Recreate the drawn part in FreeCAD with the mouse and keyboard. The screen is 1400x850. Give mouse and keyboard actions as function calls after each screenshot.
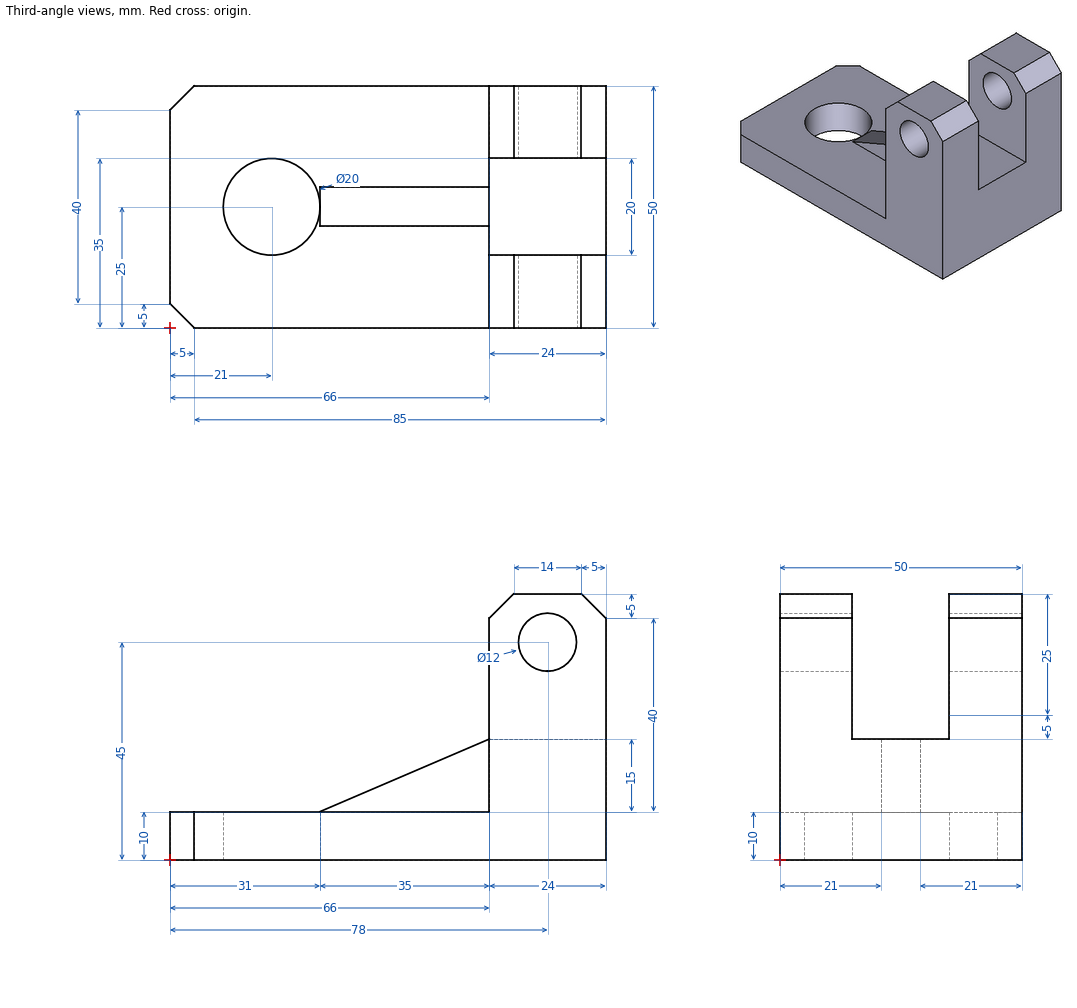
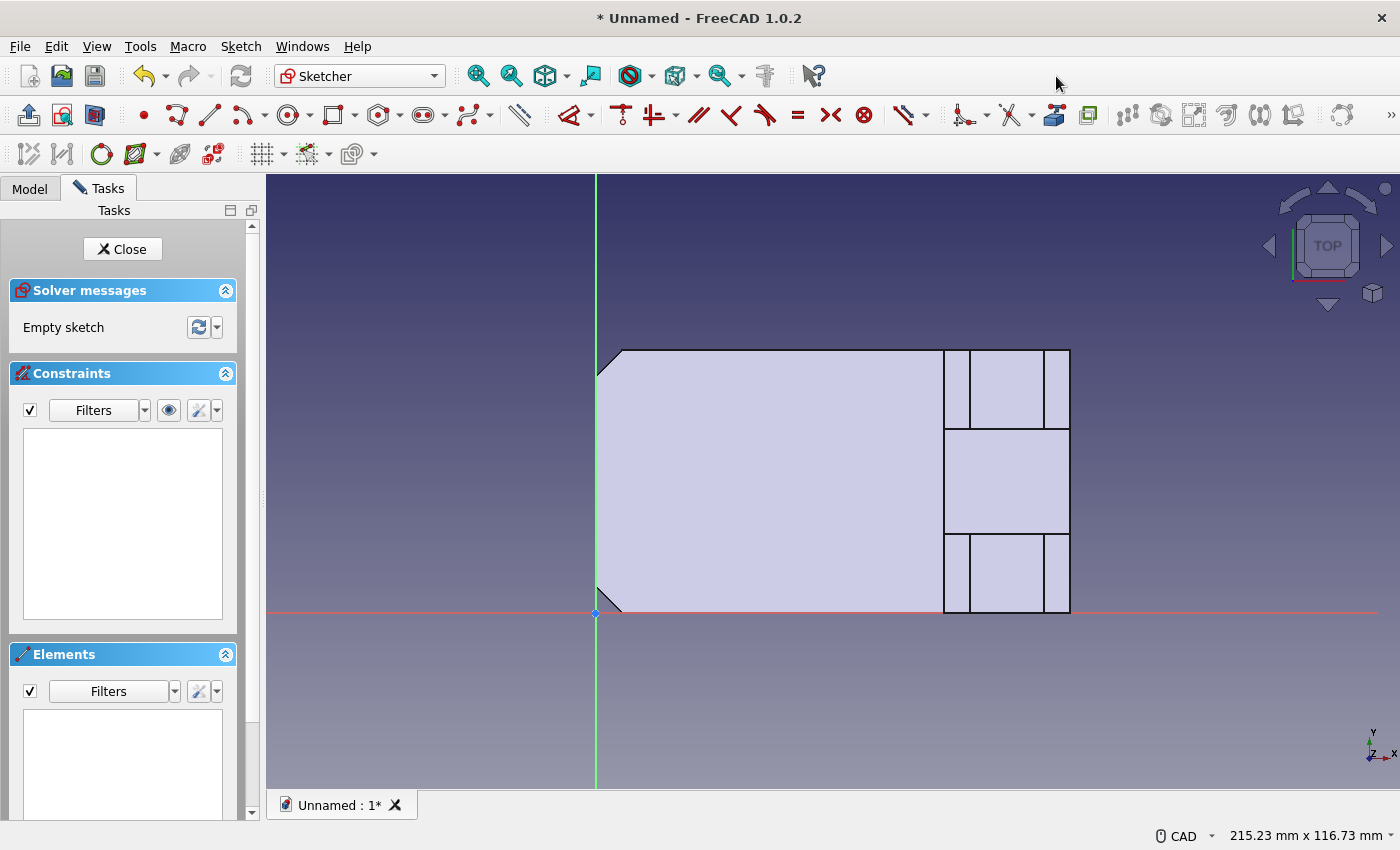
click(95, 116)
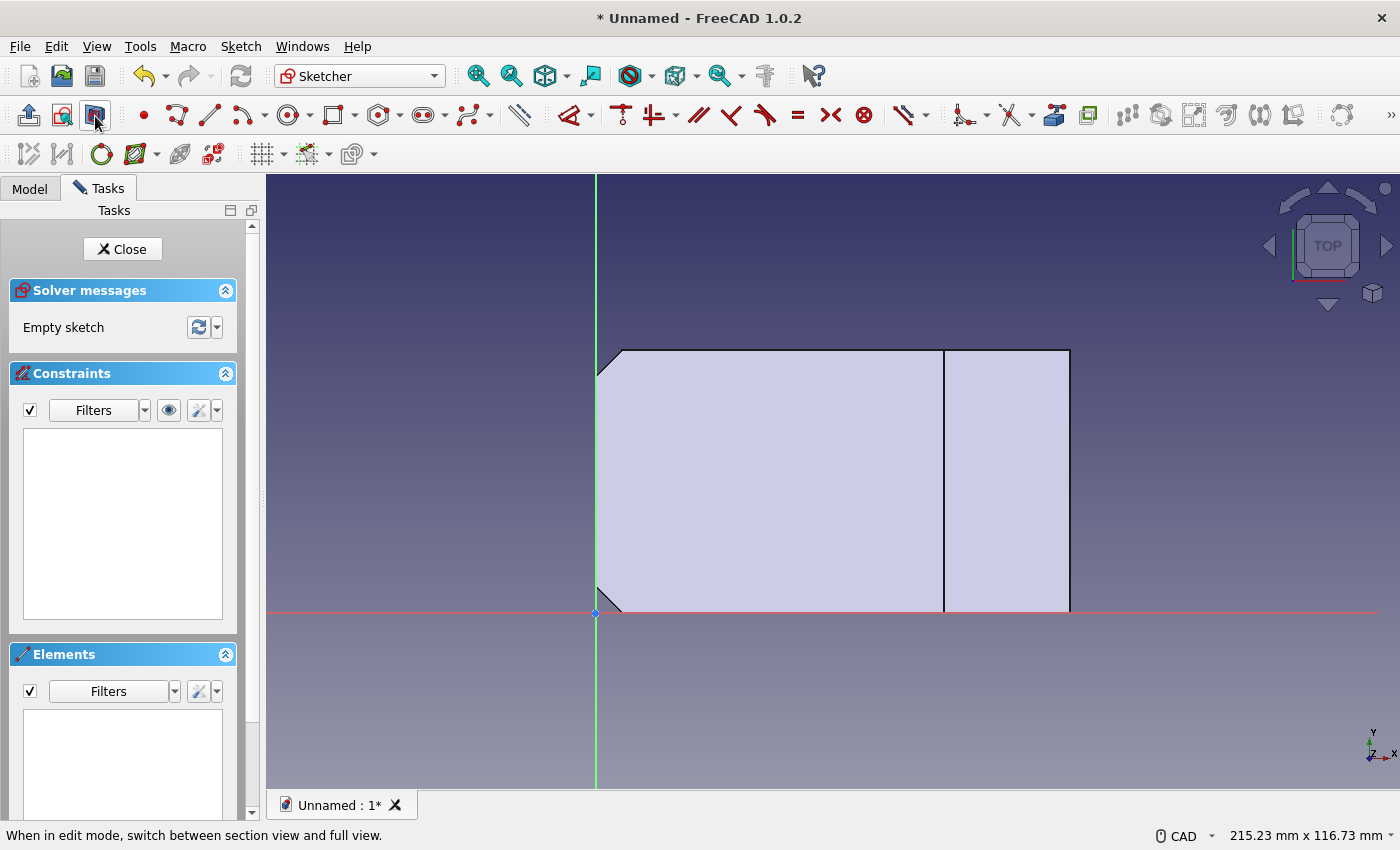
scroll(607, 553, up, 4)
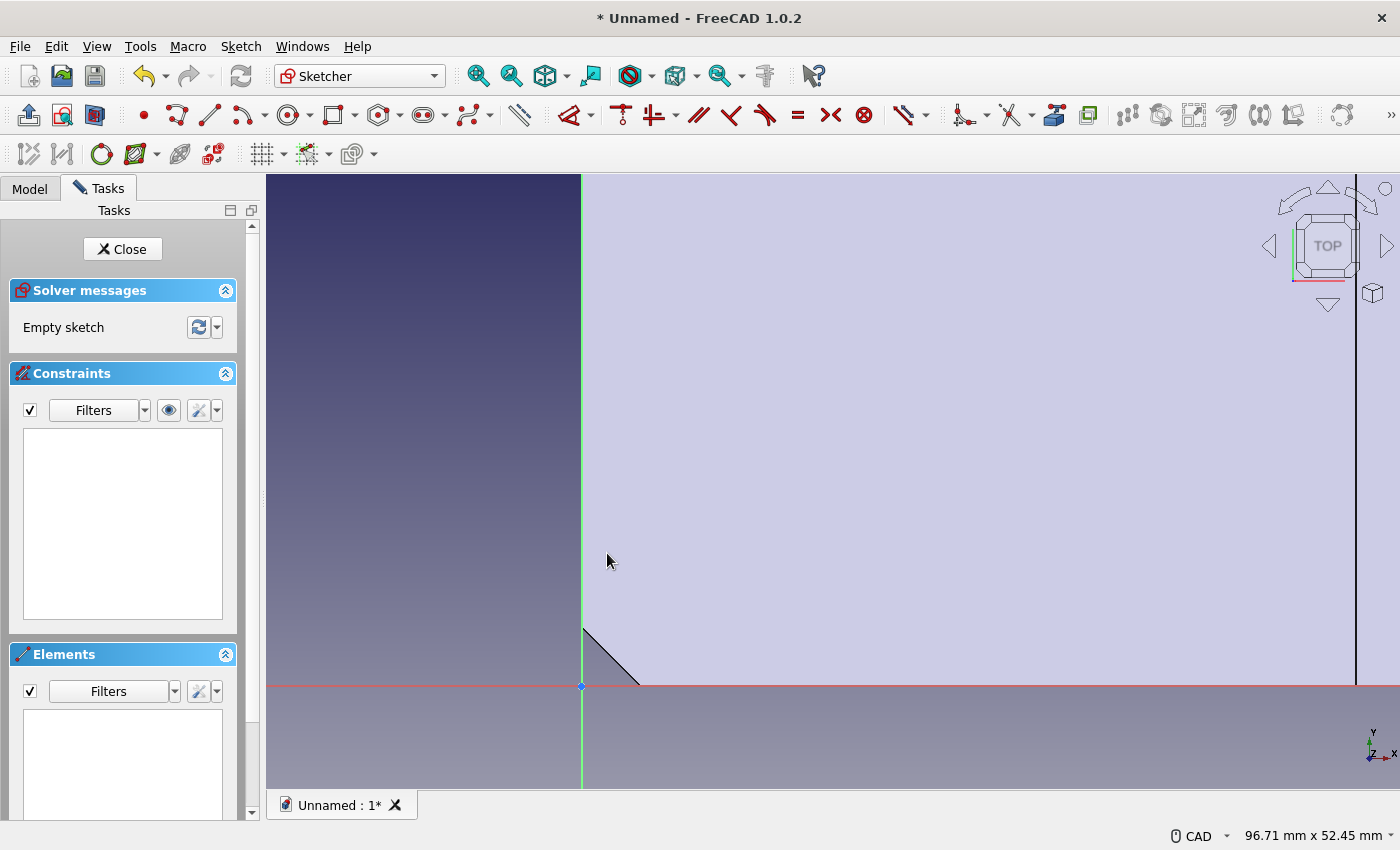
click(288, 116)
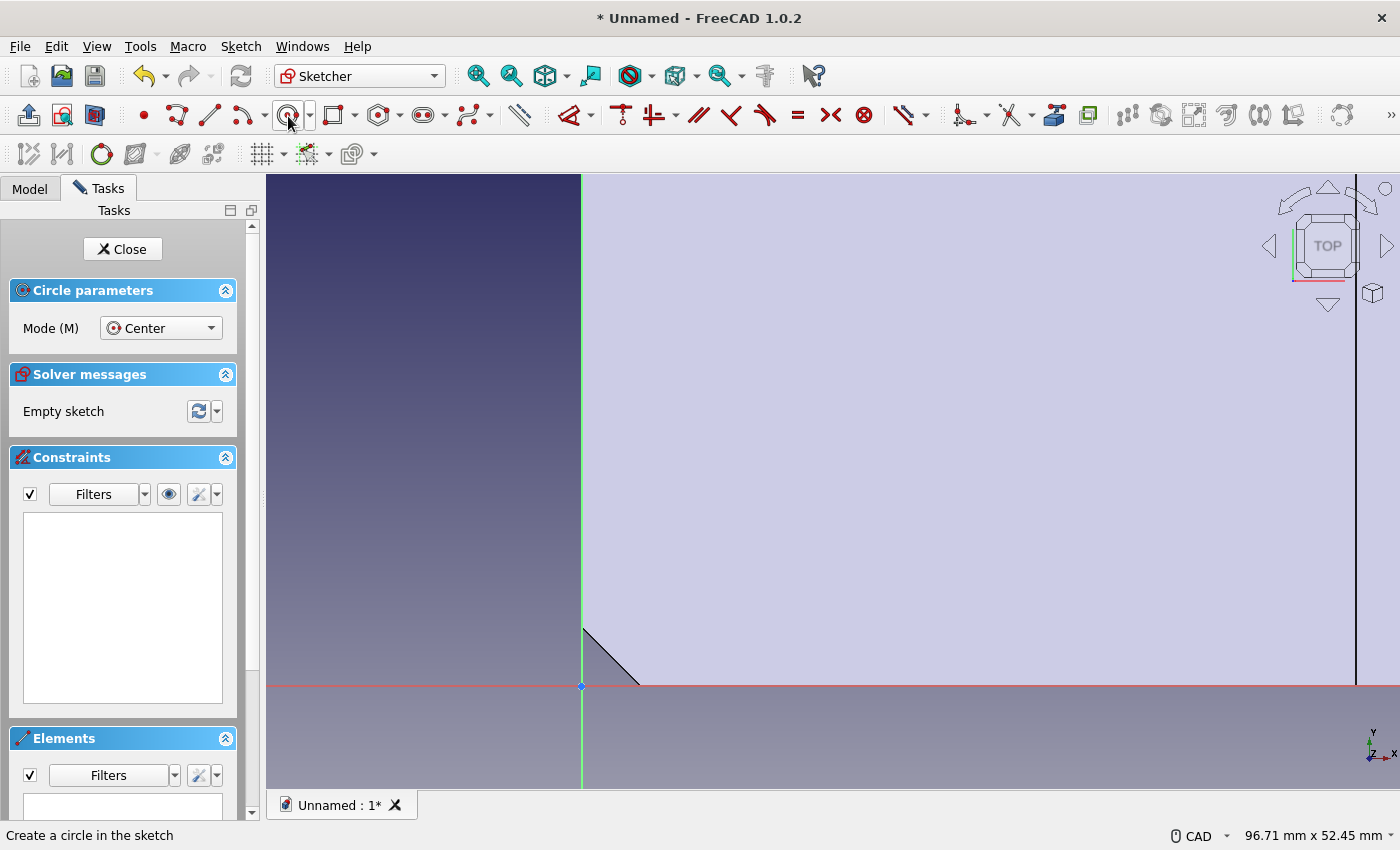
click(828, 393)
move(911, 310)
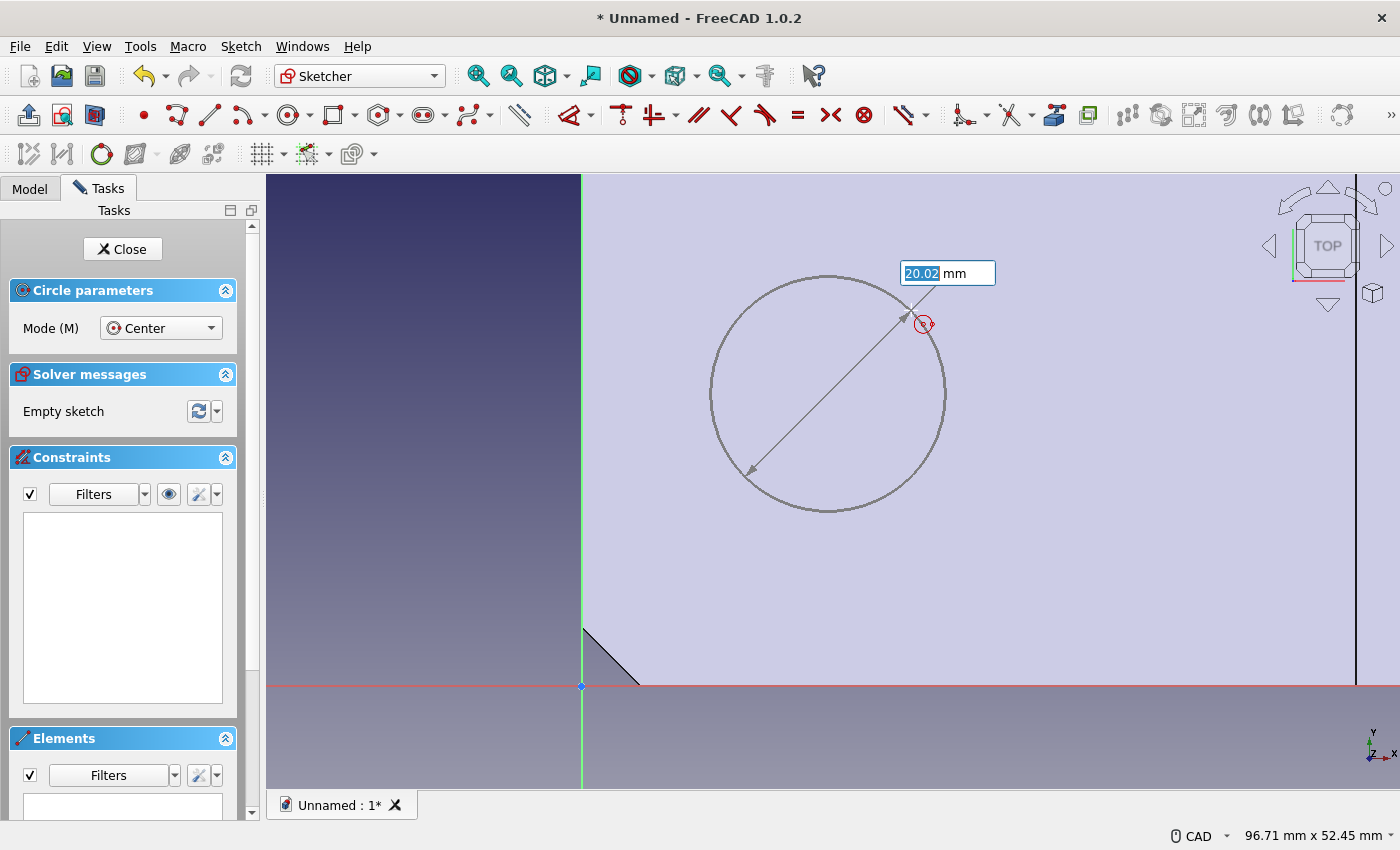
text(20)
key(Return)
key(Escape)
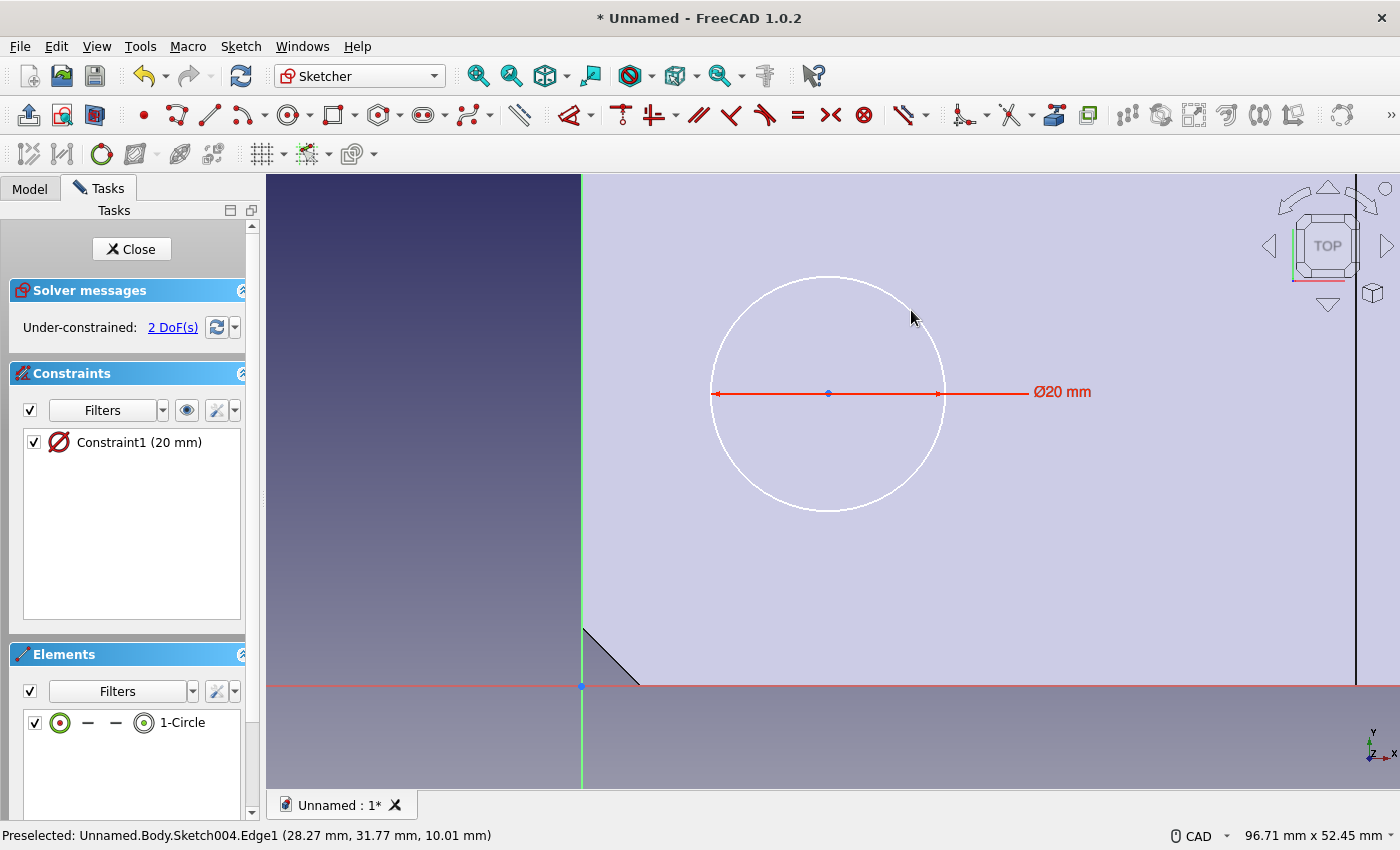
click(568, 116)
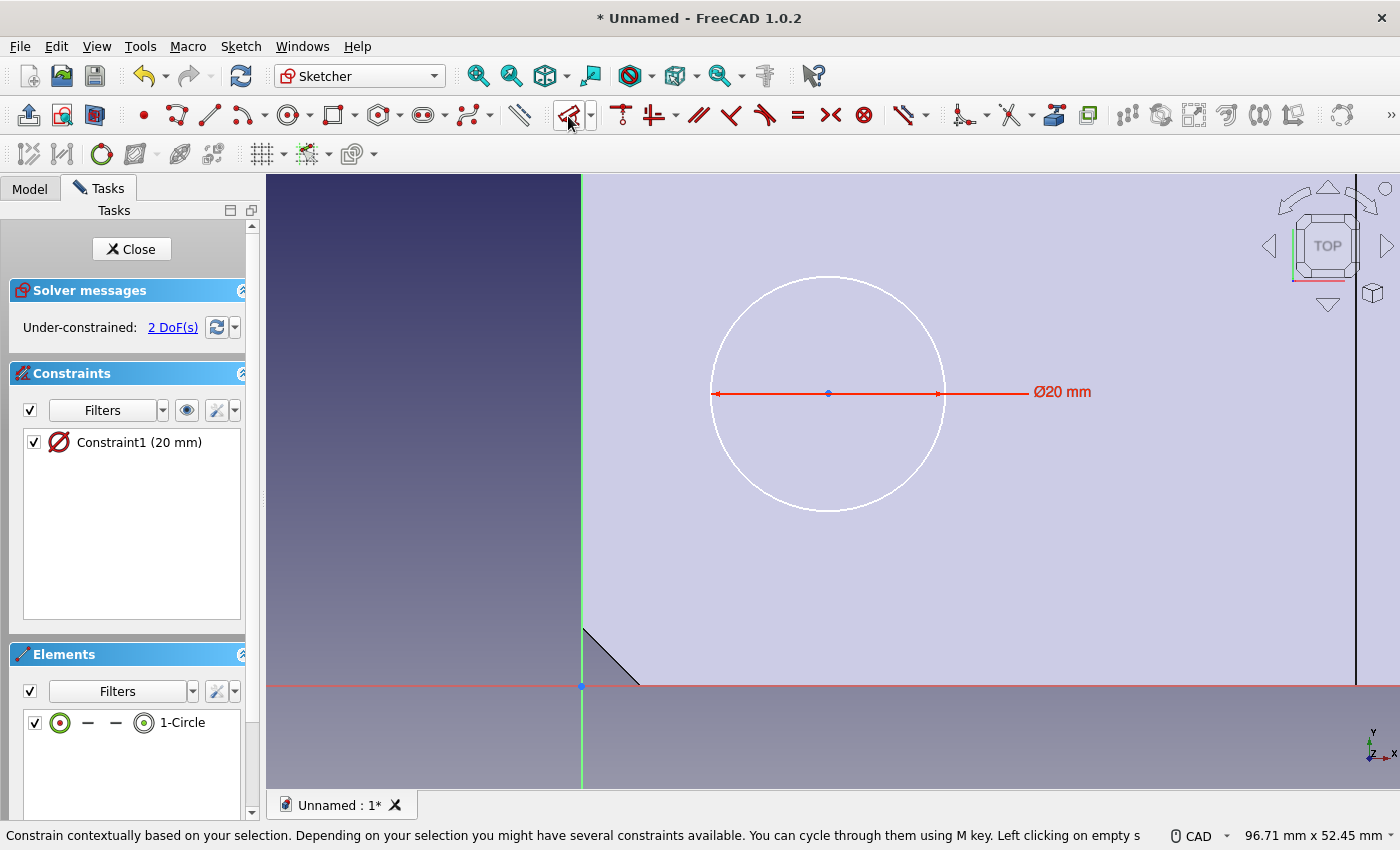
click(828, 394)
click(705, 720)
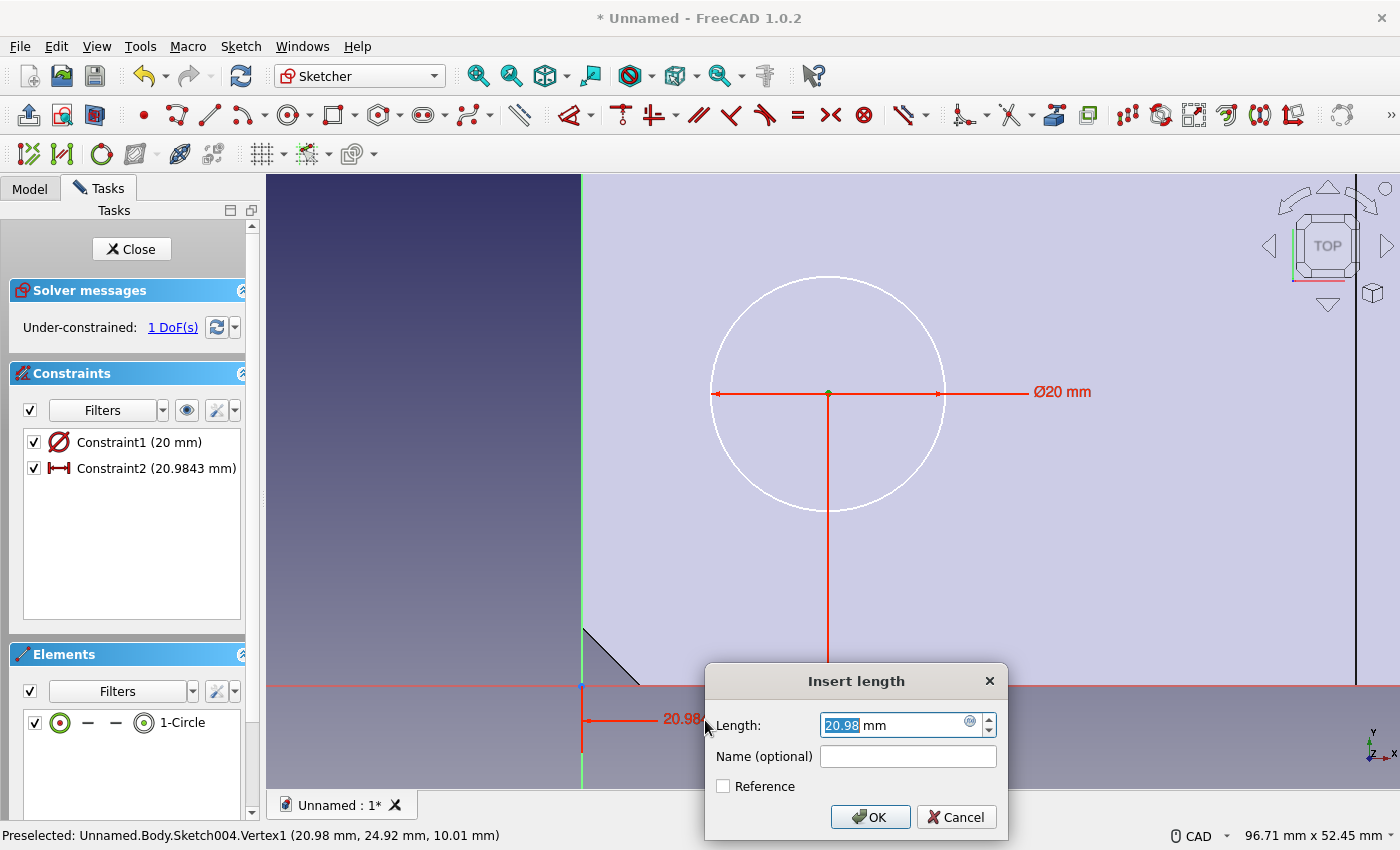
text(21)
key(Return)